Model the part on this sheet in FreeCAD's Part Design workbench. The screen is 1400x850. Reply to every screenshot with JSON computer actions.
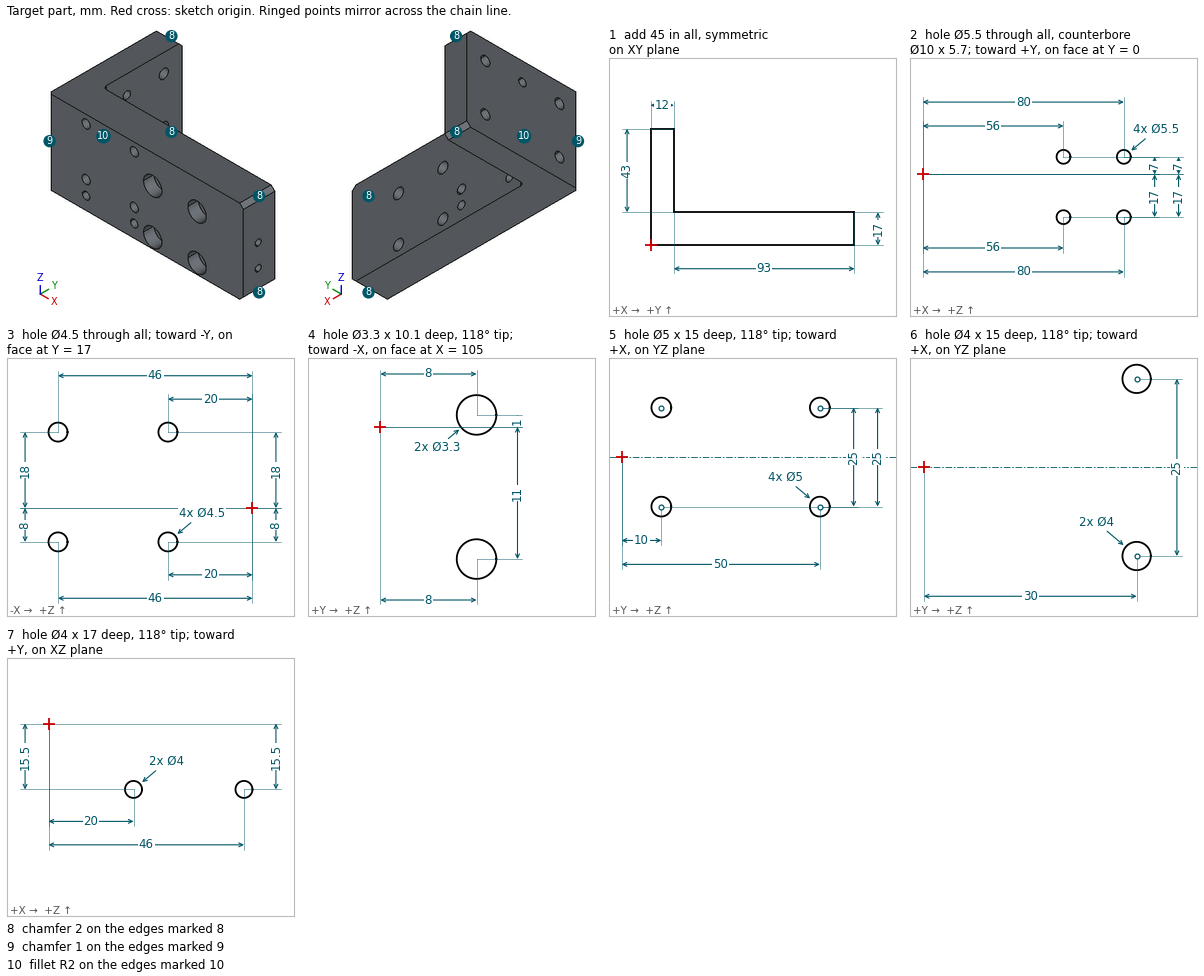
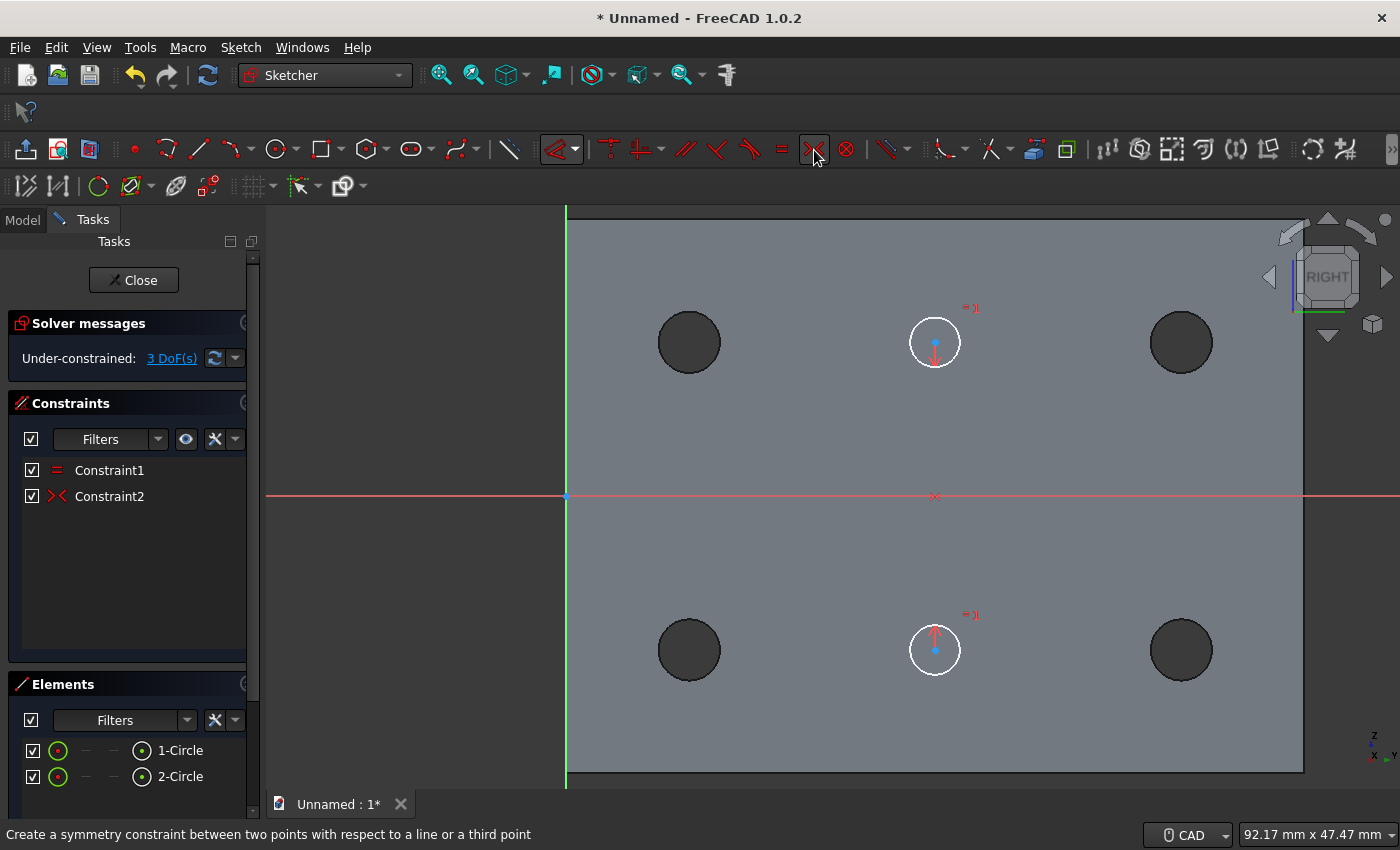
{"action": "left_click", "coordinate": [952, 632]}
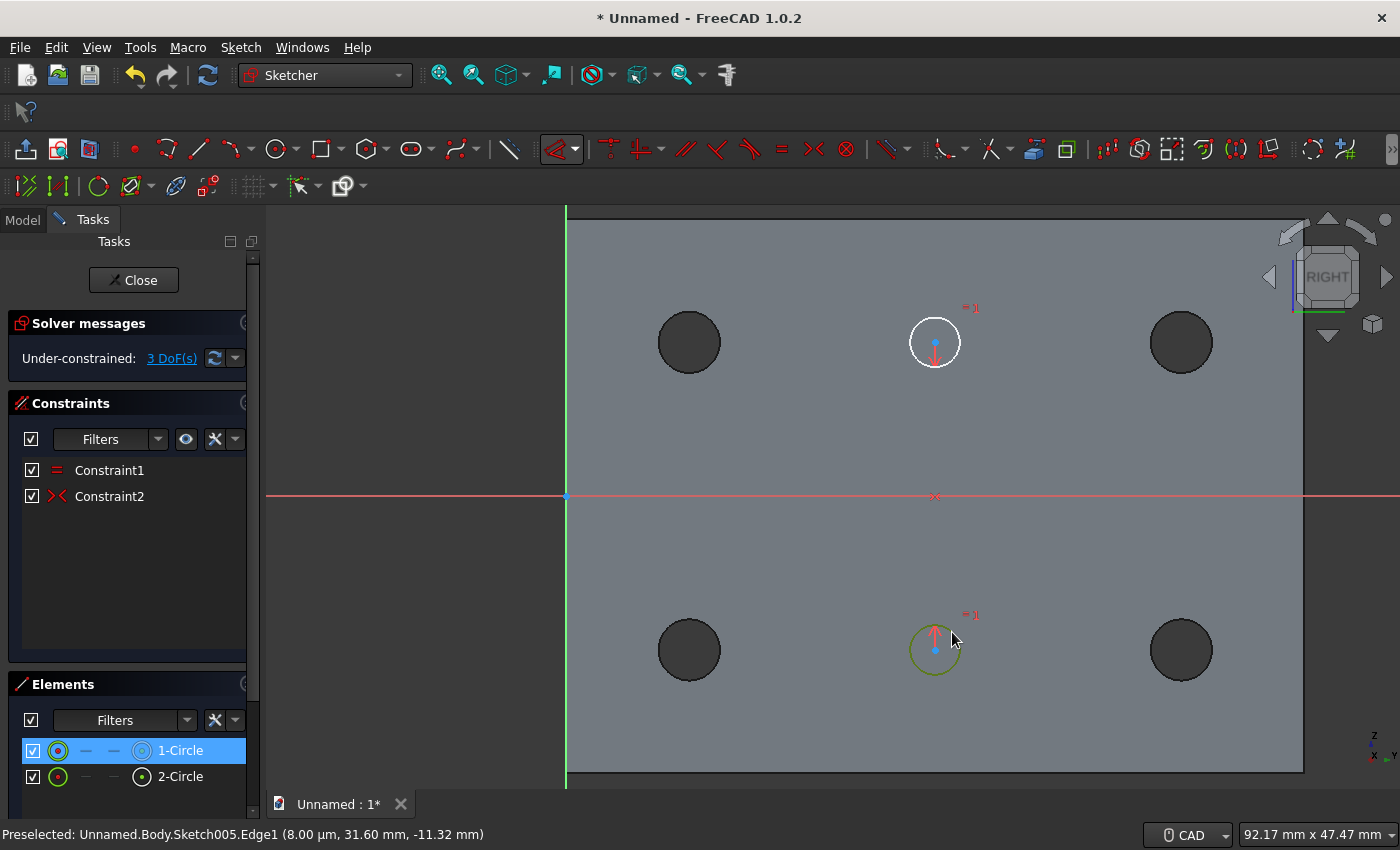
{"action": "key", "text": "k o"}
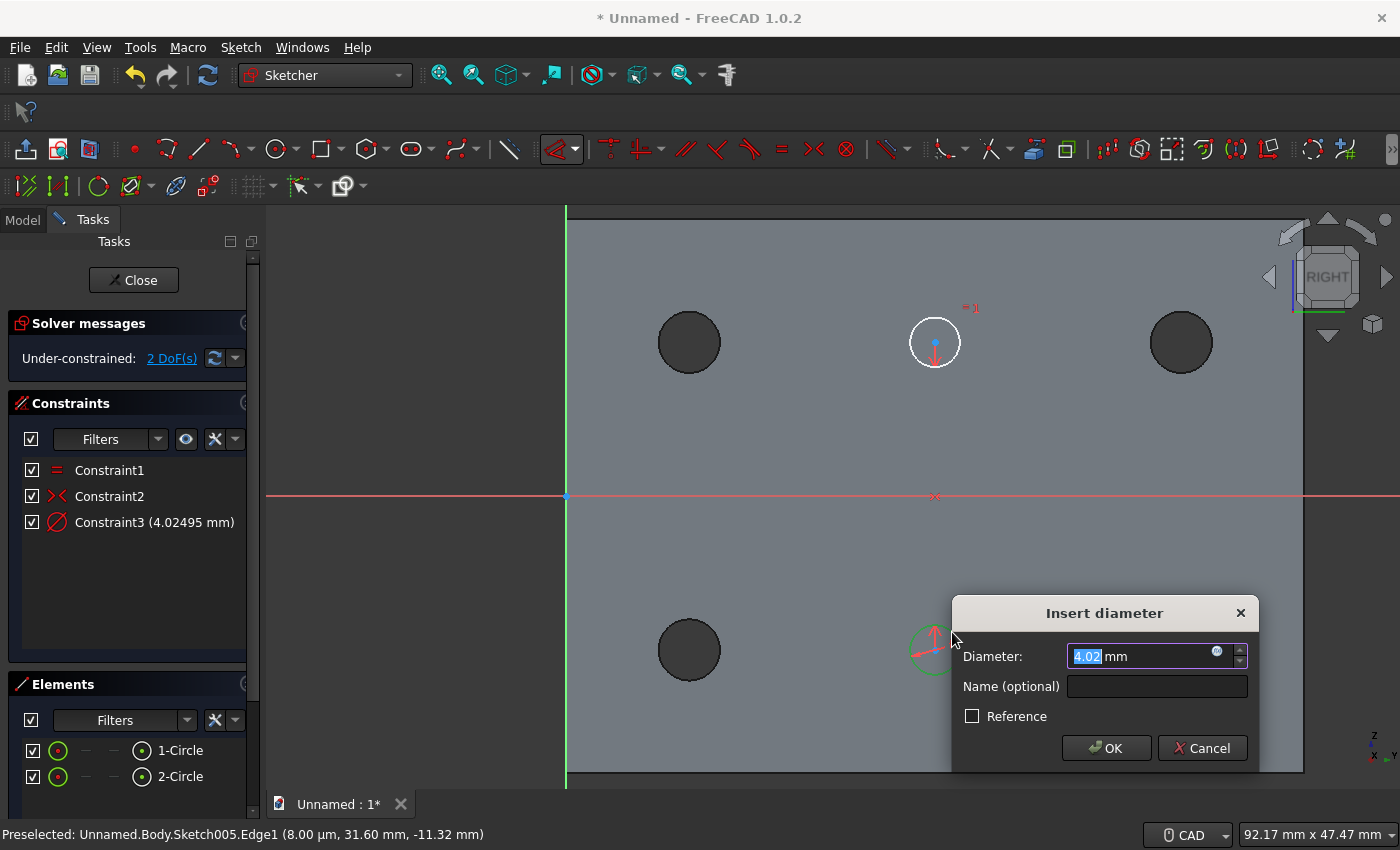
{"action": "type", "text": "4"}
{"action": "key", "text": "Return"}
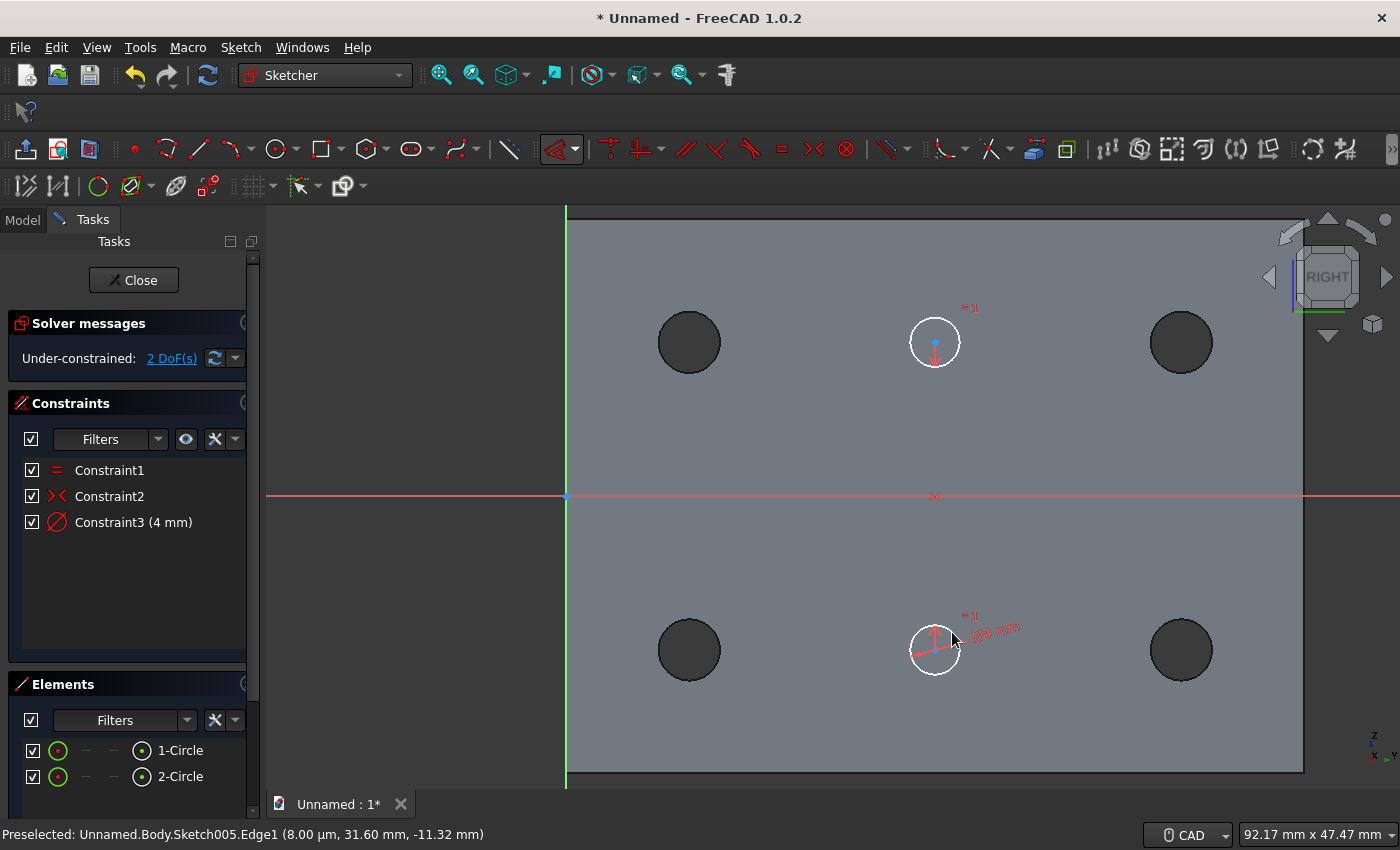
{"action": "left_click", "coordinate": [935, 650]}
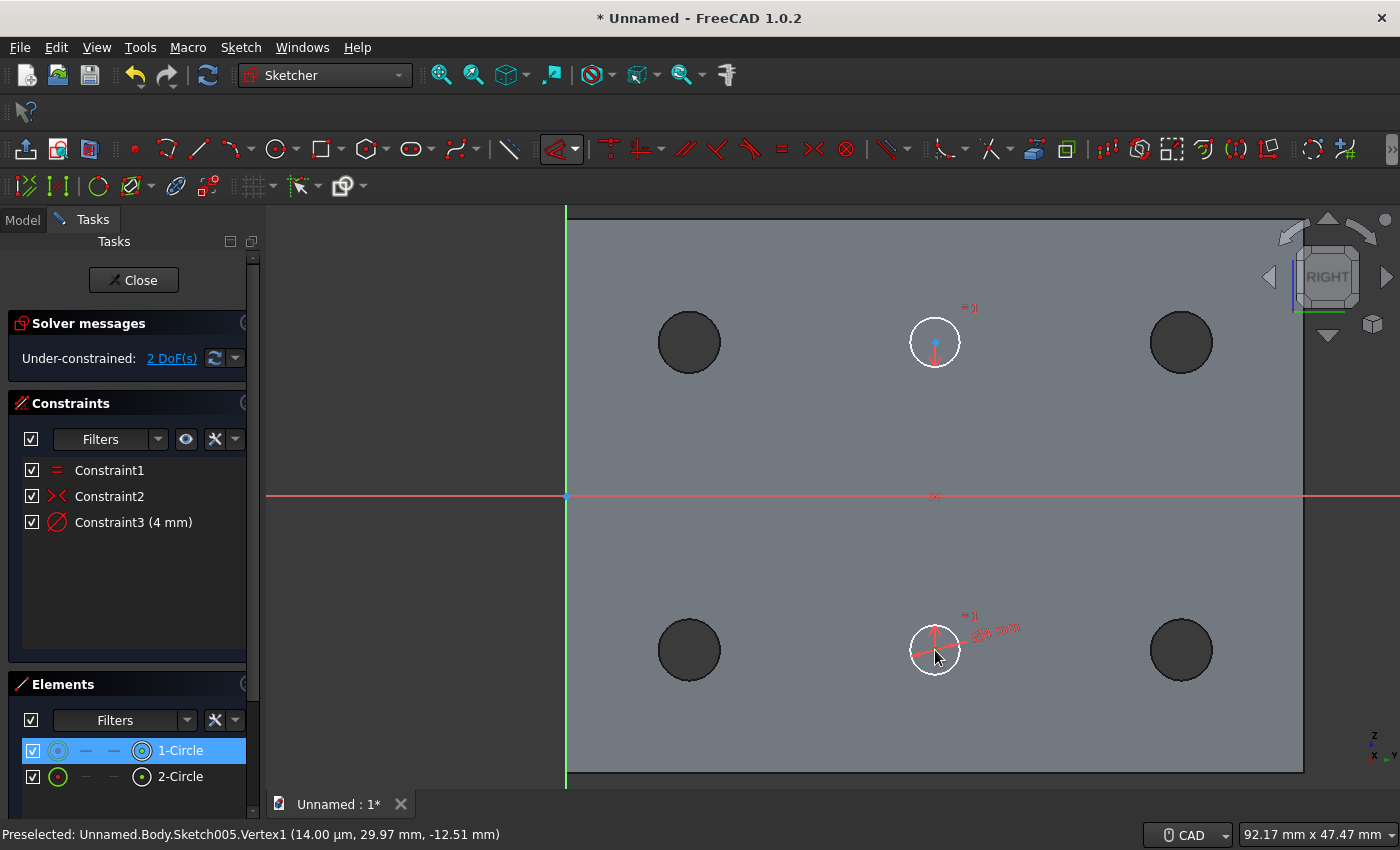
{"action": "key", "text": "l"}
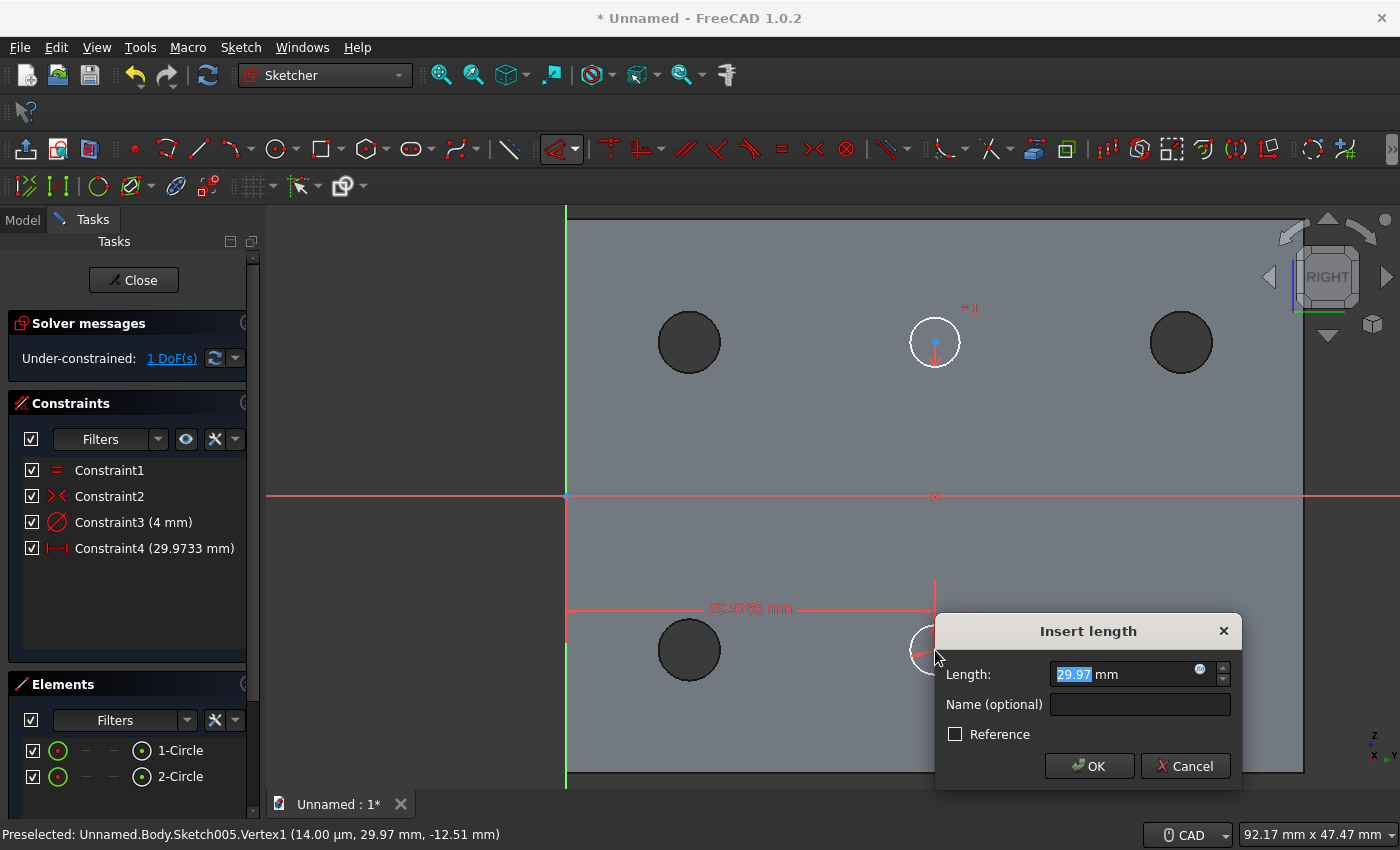
{"action": "type", "text": "30"}
{"action": "key", "text": "Return"}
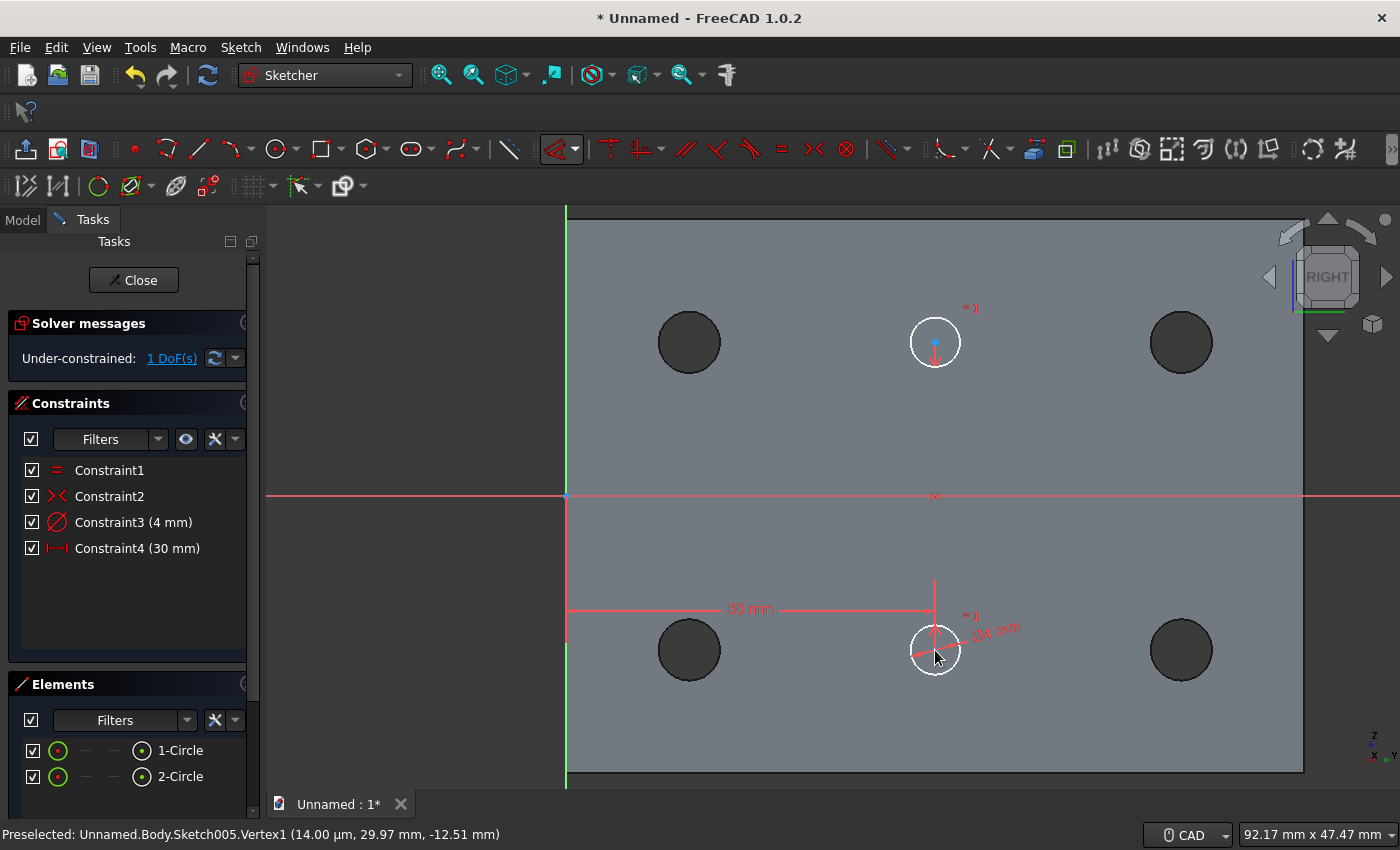
{"action": "left_click", "coordinate": [935, 650]}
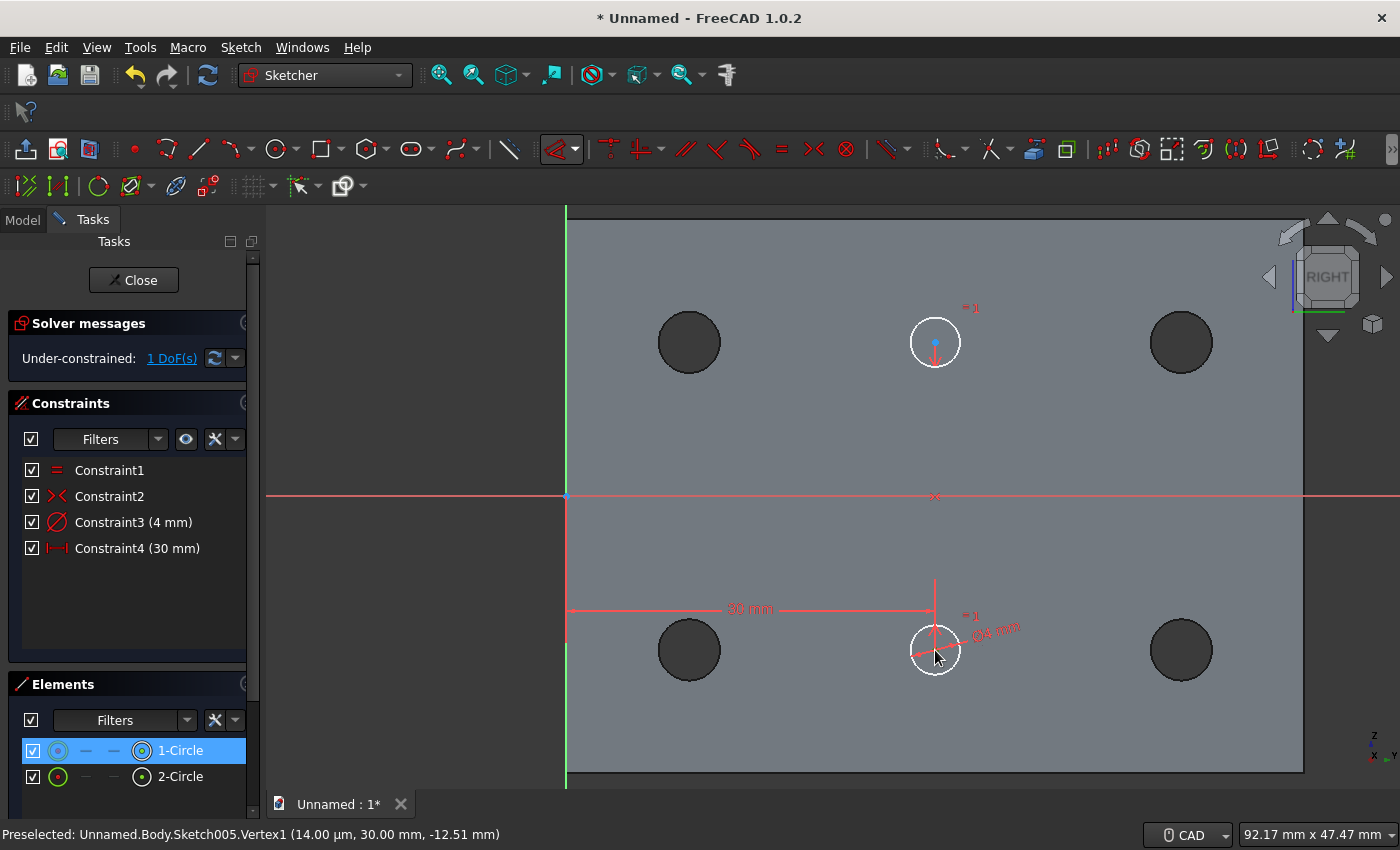
{"action": "left_click", "coordinate": [935, 342]}